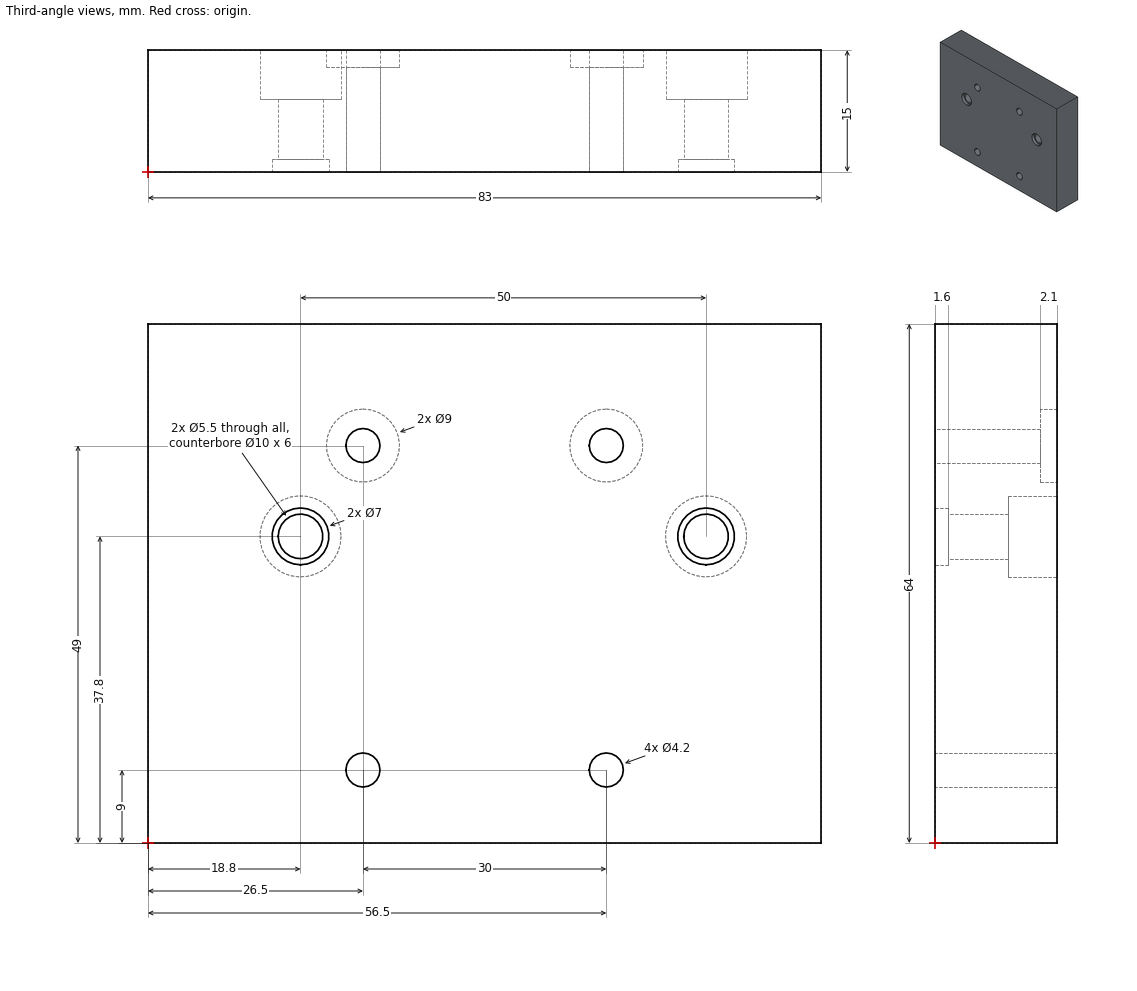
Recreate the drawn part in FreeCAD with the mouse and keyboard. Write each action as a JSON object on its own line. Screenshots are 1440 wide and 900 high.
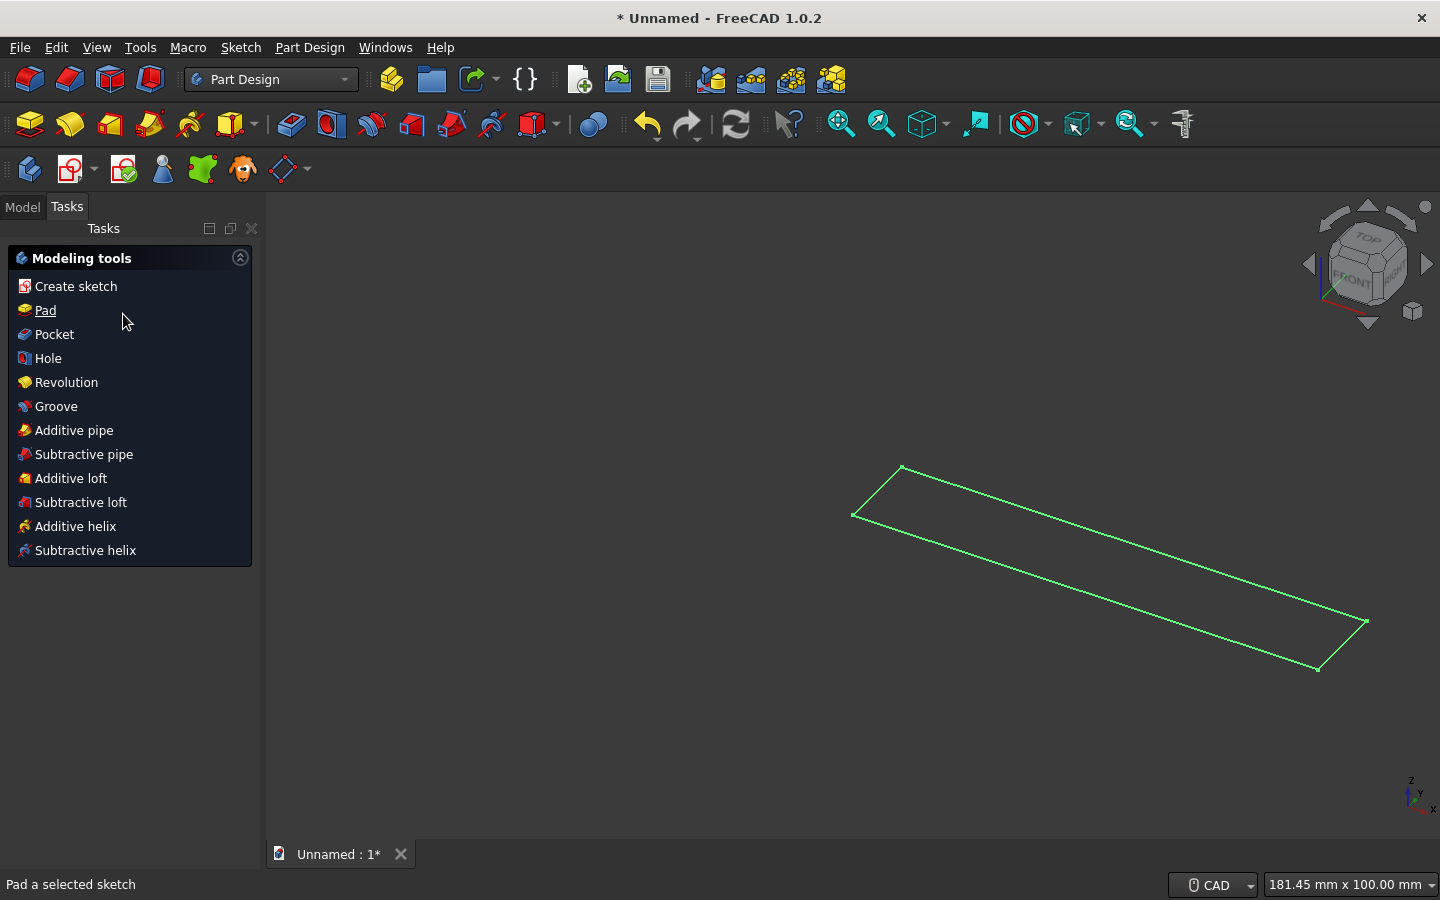
{"action": "left_click", "coordinate": [30, 124]}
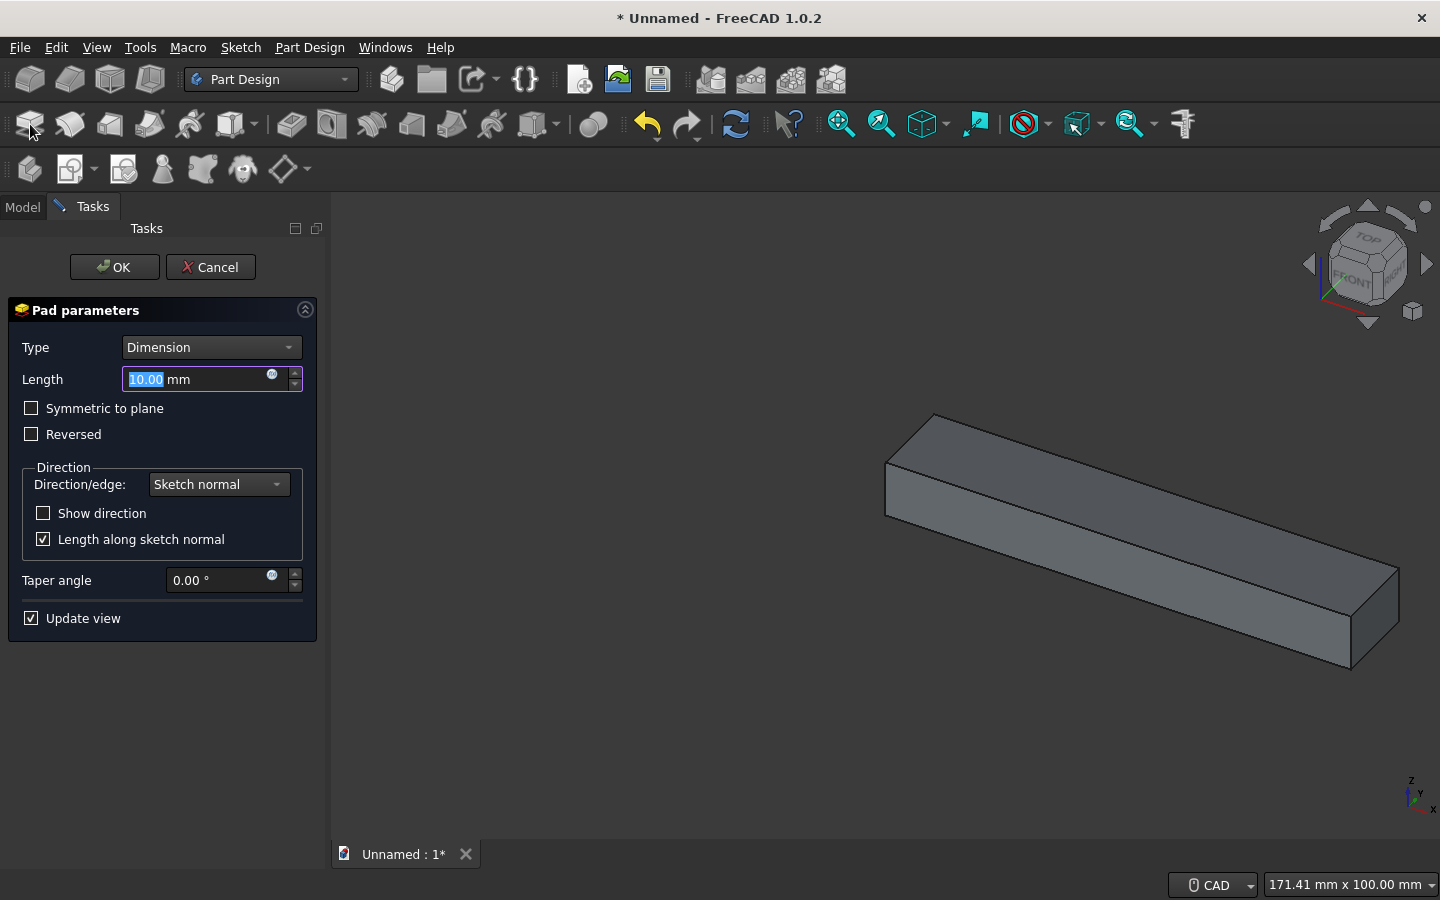
{"action": "type", "text": "64"}
{"action": "key", "text": "Tab"}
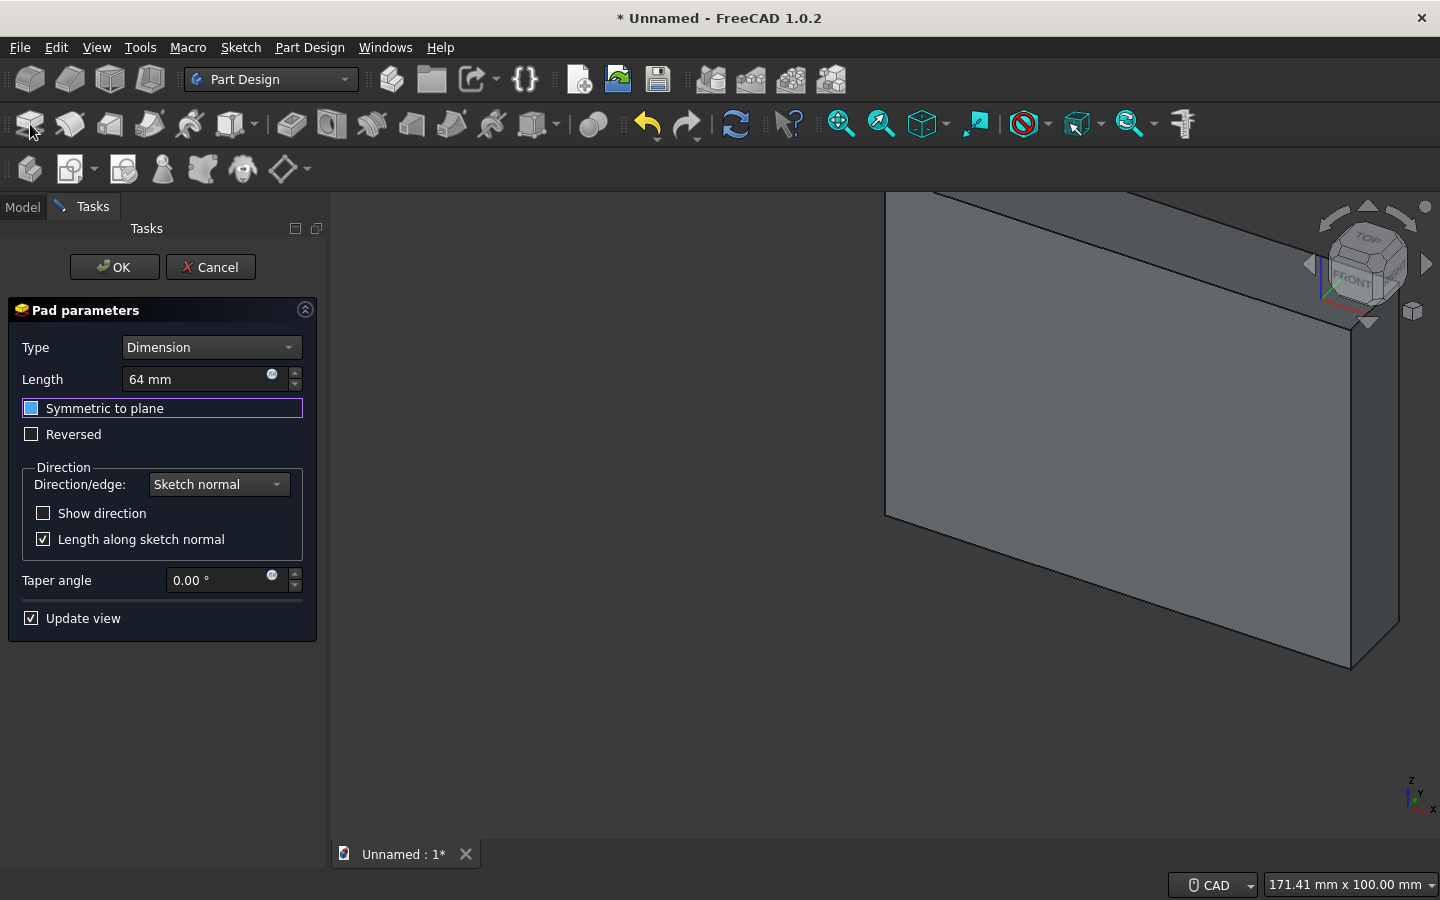
{"action": "left_click", "coordinate": [115, 267]}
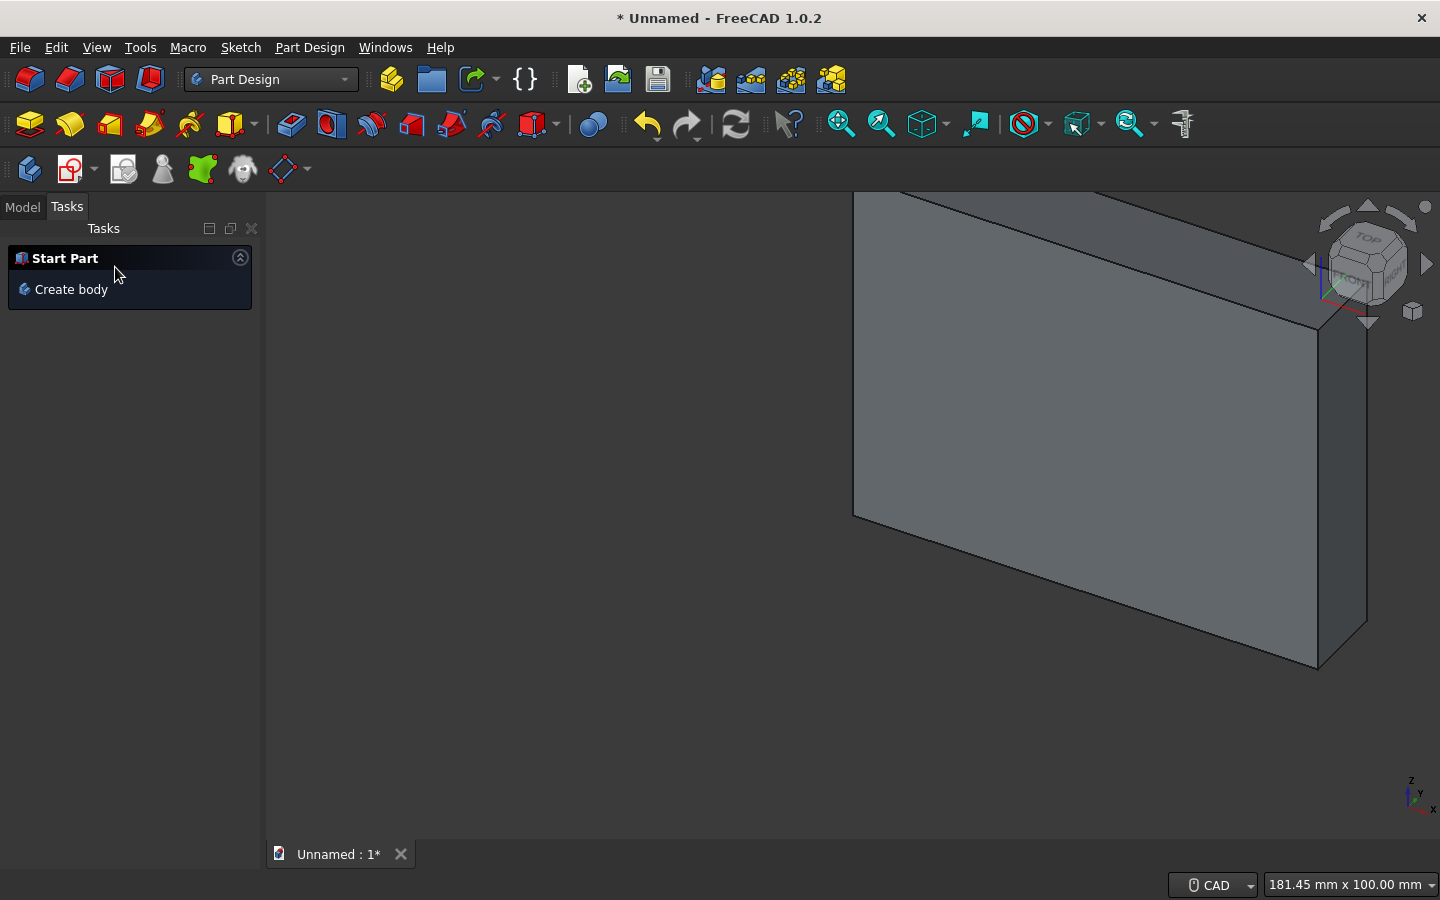
{"action": "left_click", "coordinate": [842, 124]}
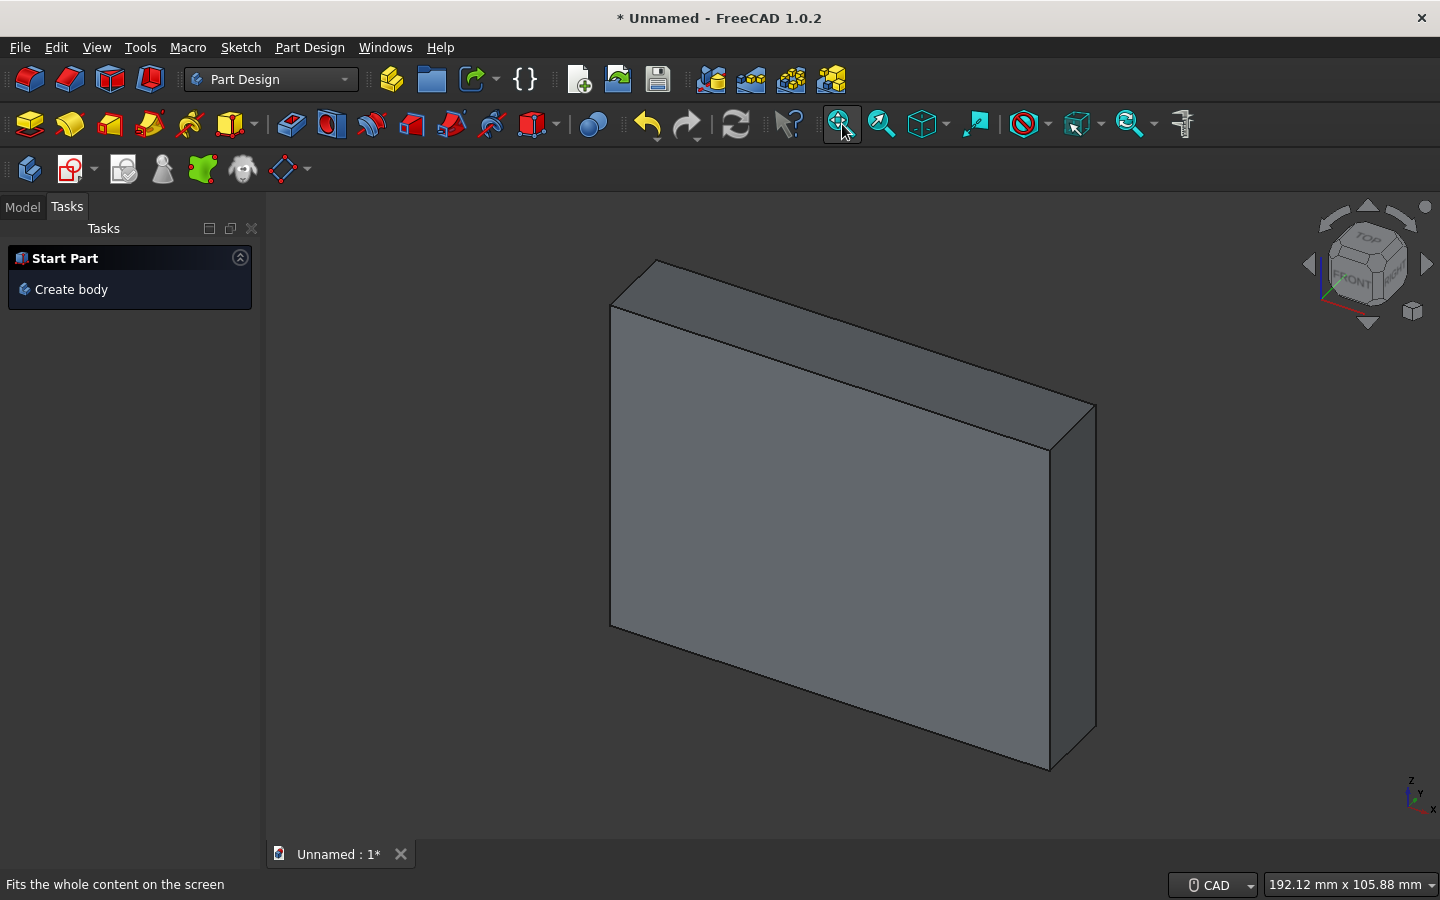
{"action": "key", "text": "4"}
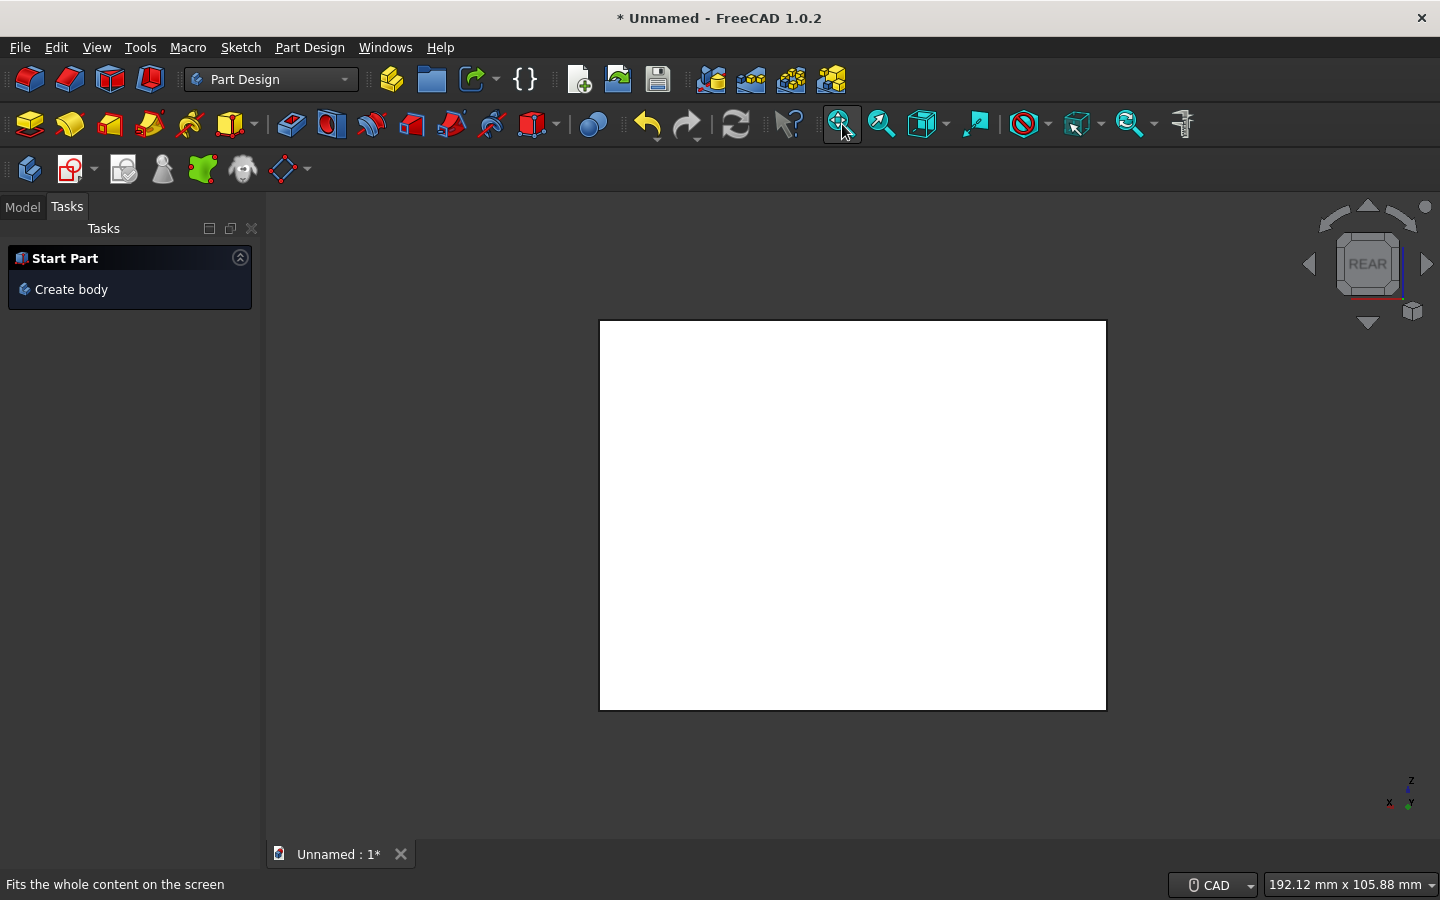
{"action": "left_click", "coordinate": [853, 515]}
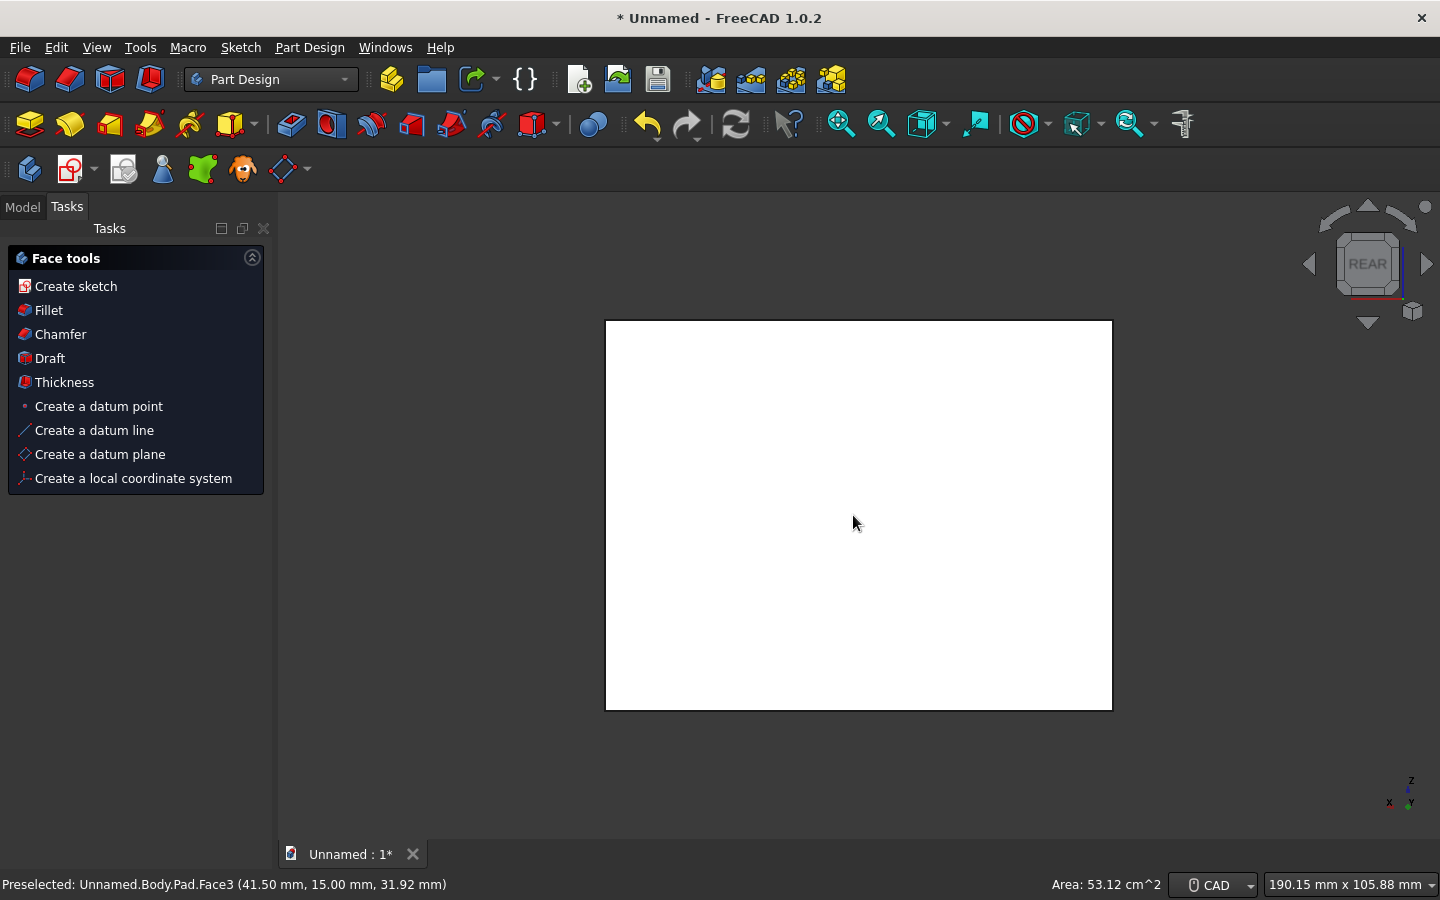
{"action": "left_click", "coordinate": [70, 170]}